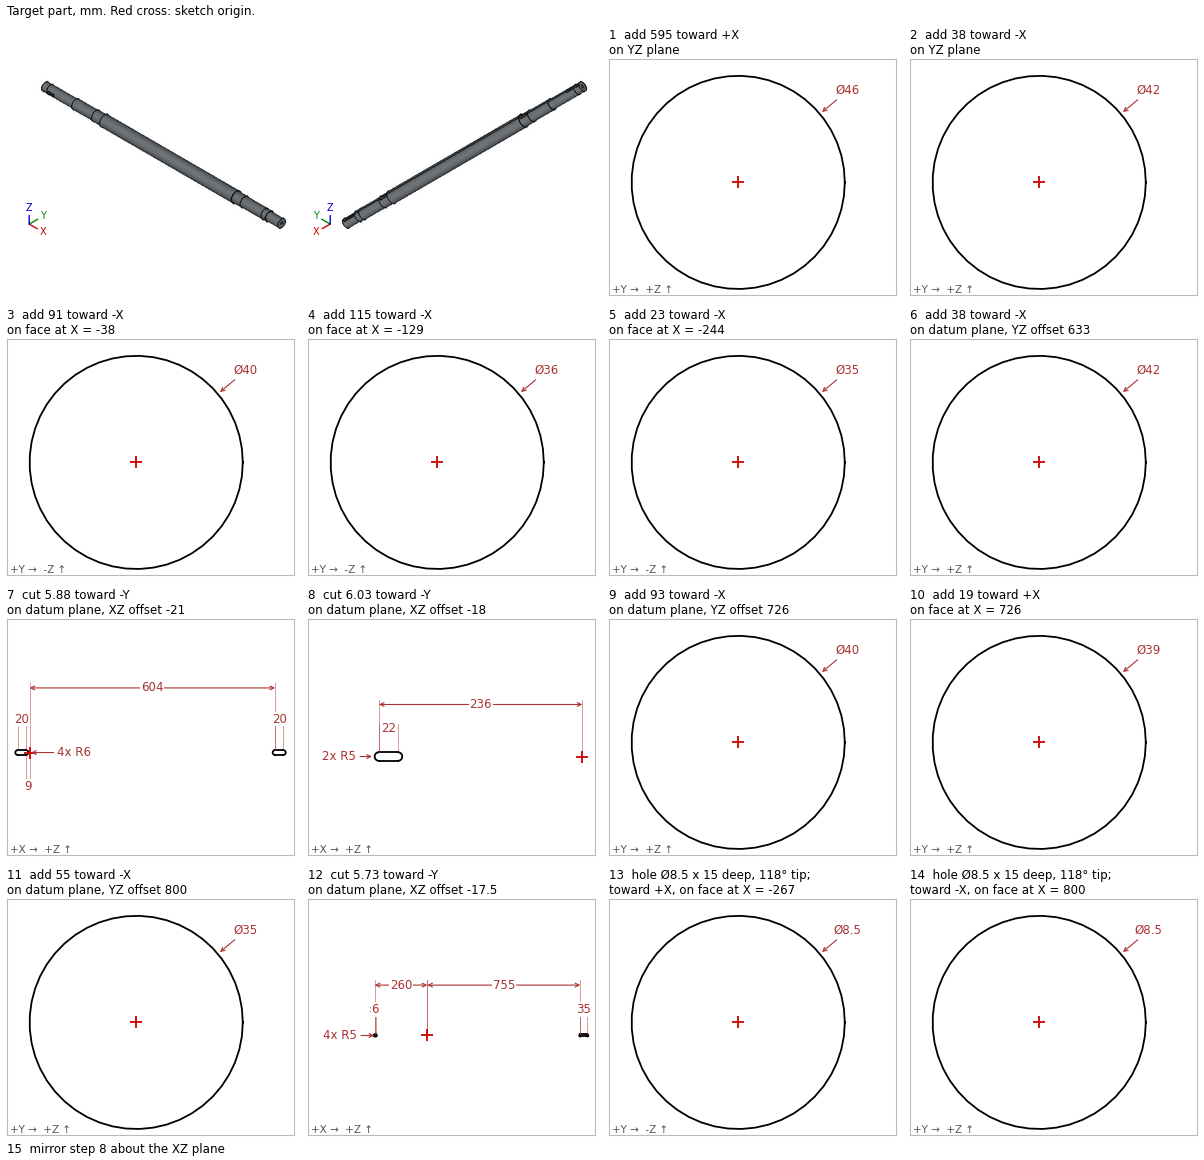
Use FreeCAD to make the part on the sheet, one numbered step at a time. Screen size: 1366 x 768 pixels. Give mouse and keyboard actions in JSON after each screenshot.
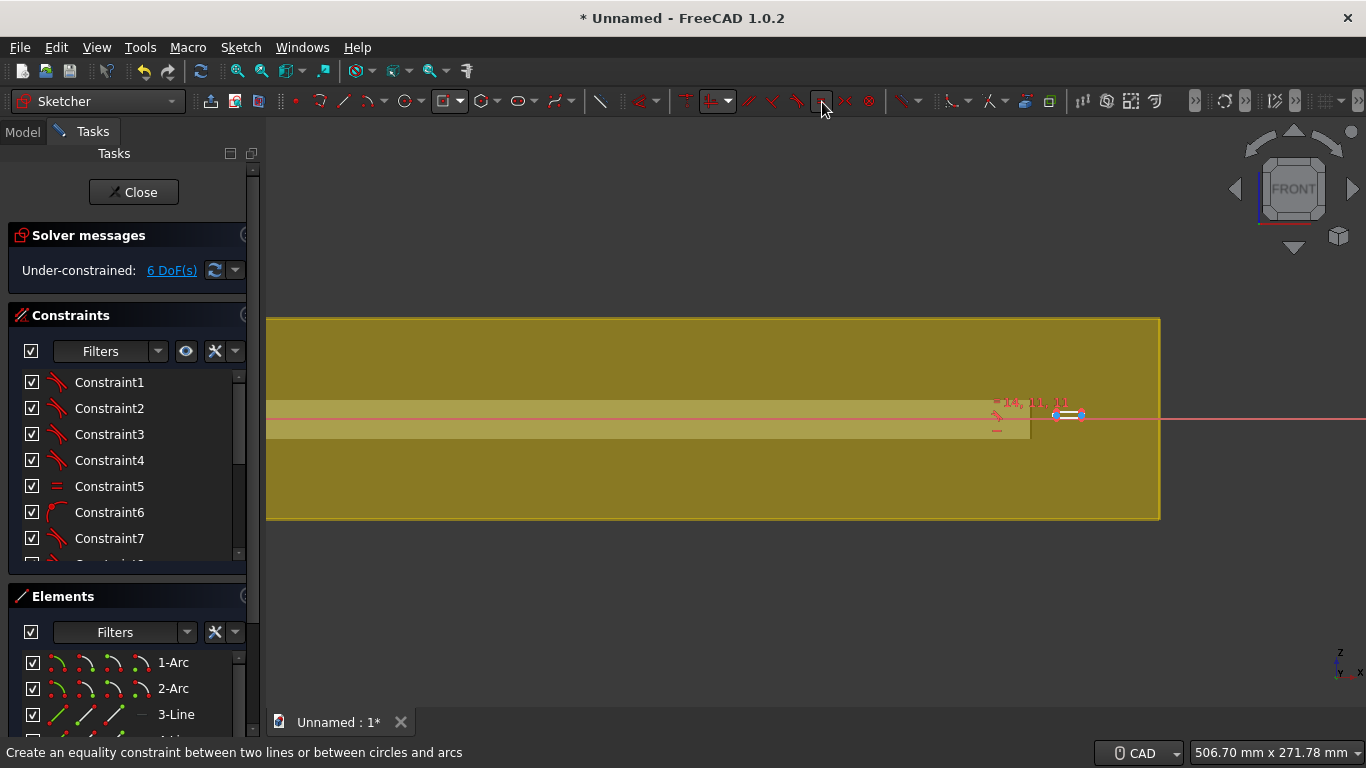
{"action": "scroll", "coordinate": [1056, 415], "scroll_direction": "up", "scroll_amount": 7}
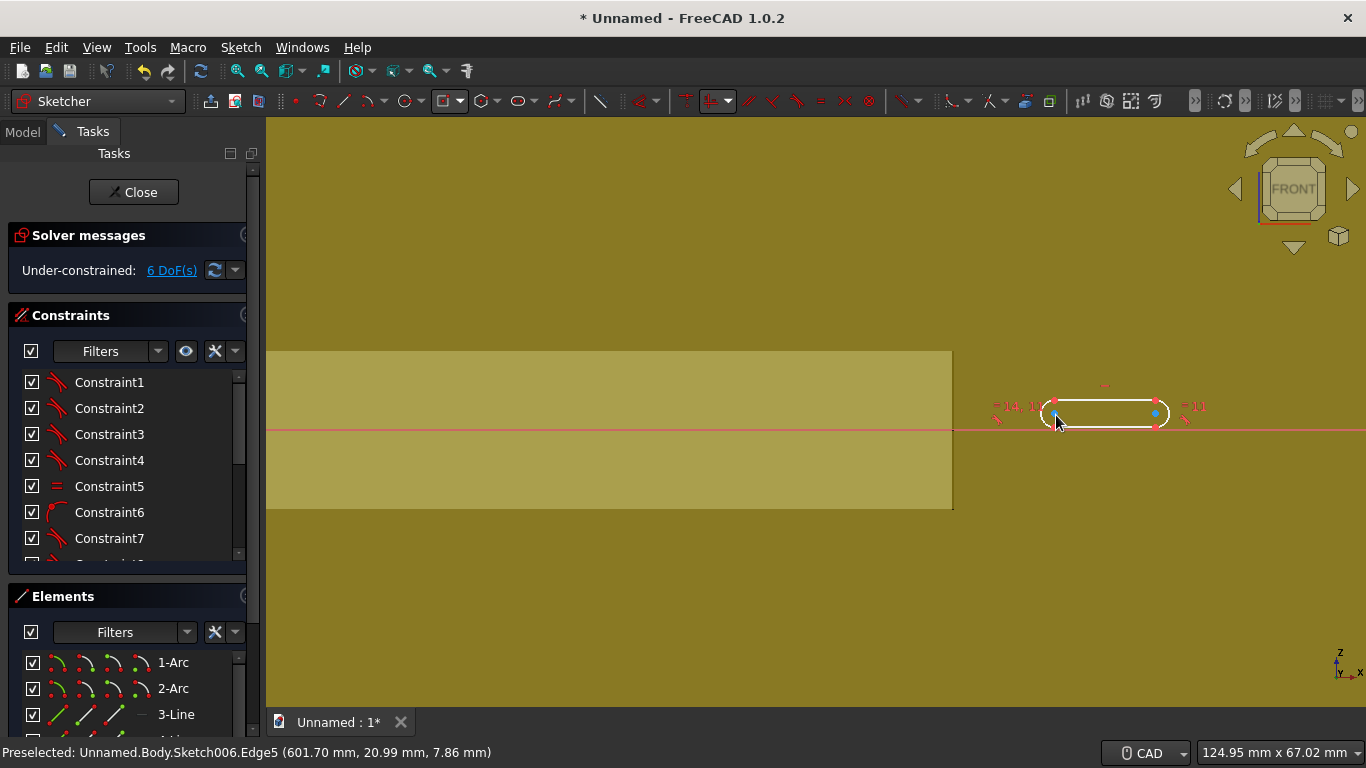
{"action": "left_click", "coordinate": [1055, 414]}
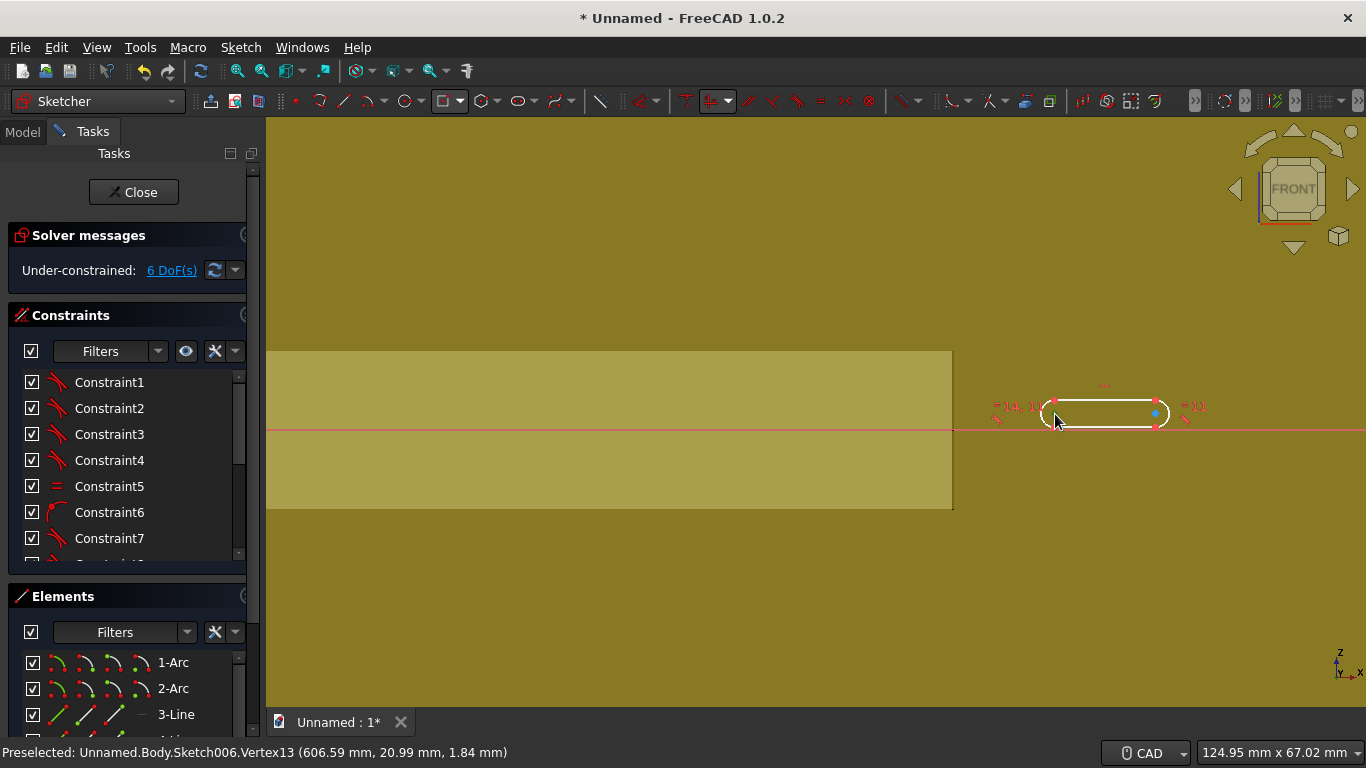
{"action": "left_click", "coordinate": [359, 430]}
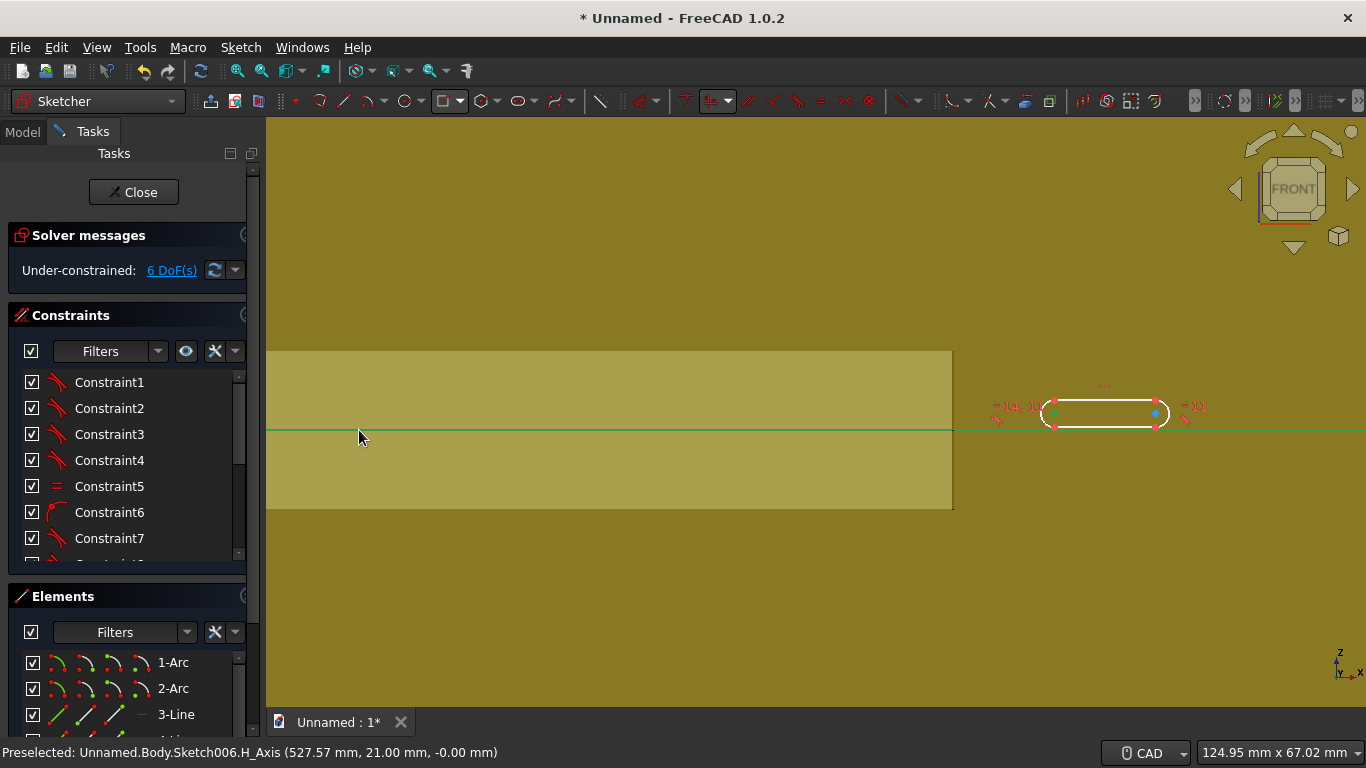
{"action": "key", "text": "c"}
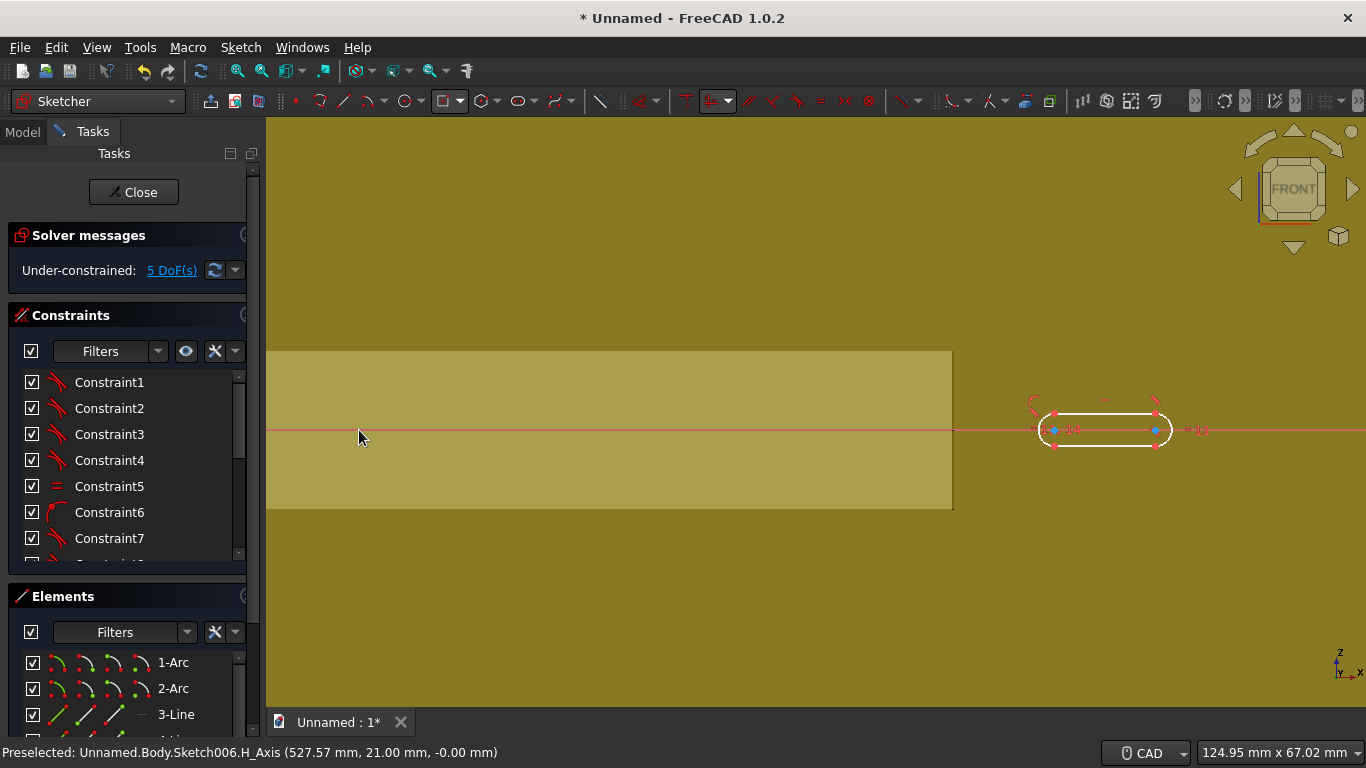
{"action": "scroll", "coordinate": [1048, 410], "scroll_direction": "down", "scroll_amount": 11}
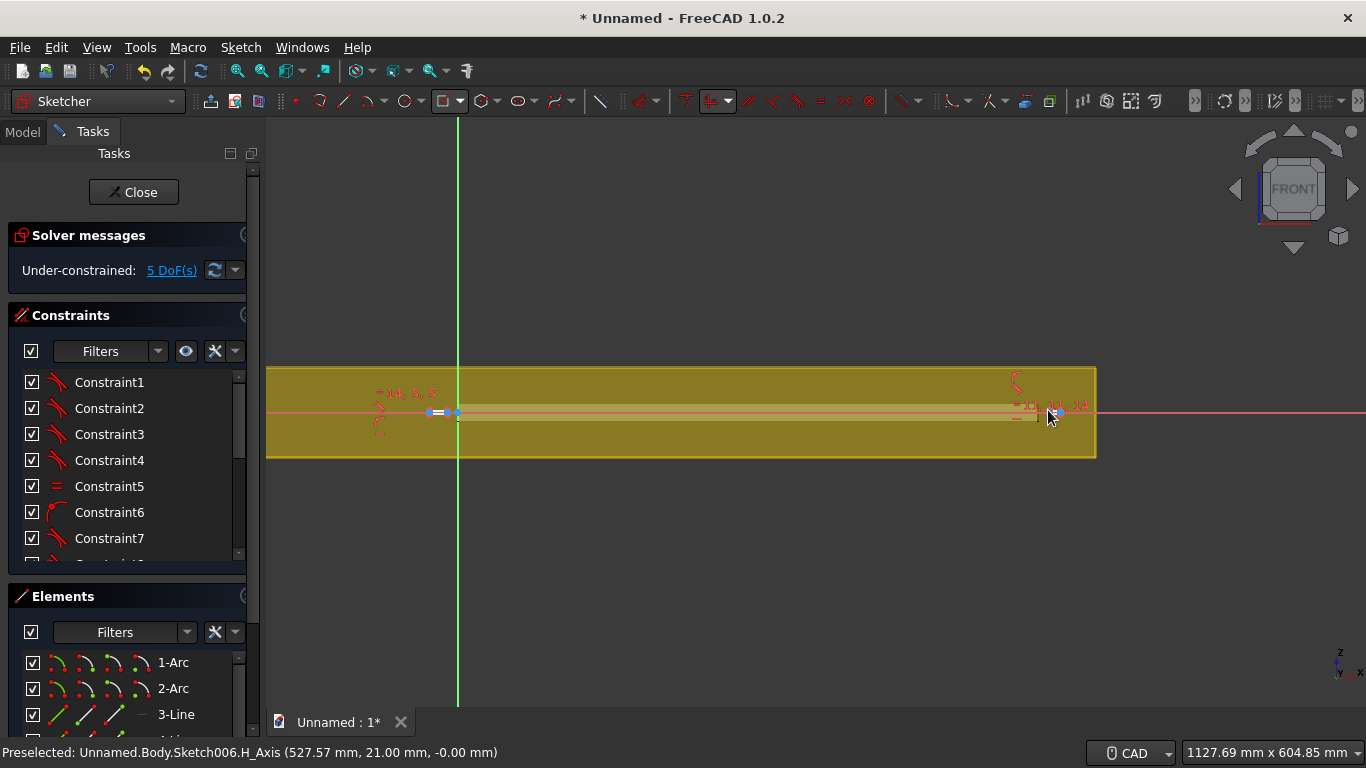
{"action": "scroll", "coordinate": [429, 412], "scroll_direction": "up", "scroll_amount": 13}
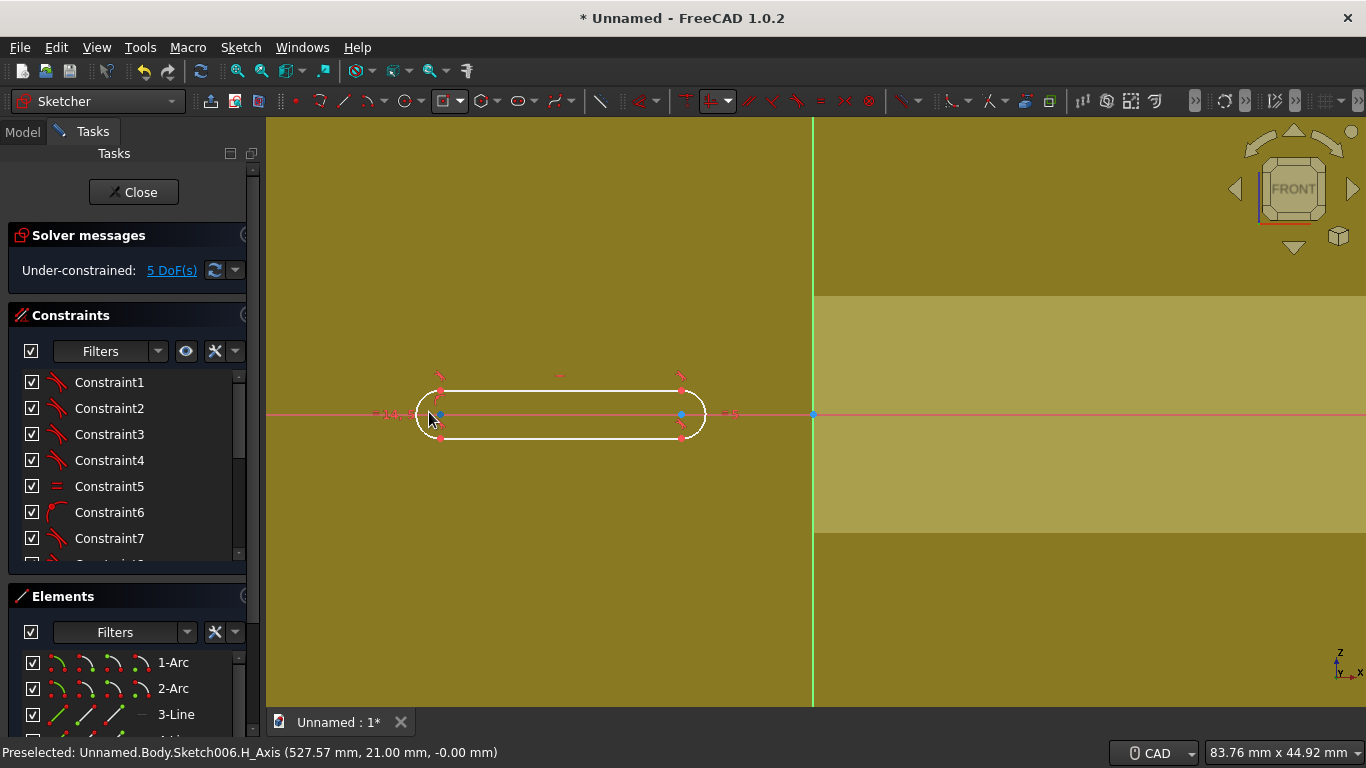
{"action": "left_click", "coordinate": [421, 401]}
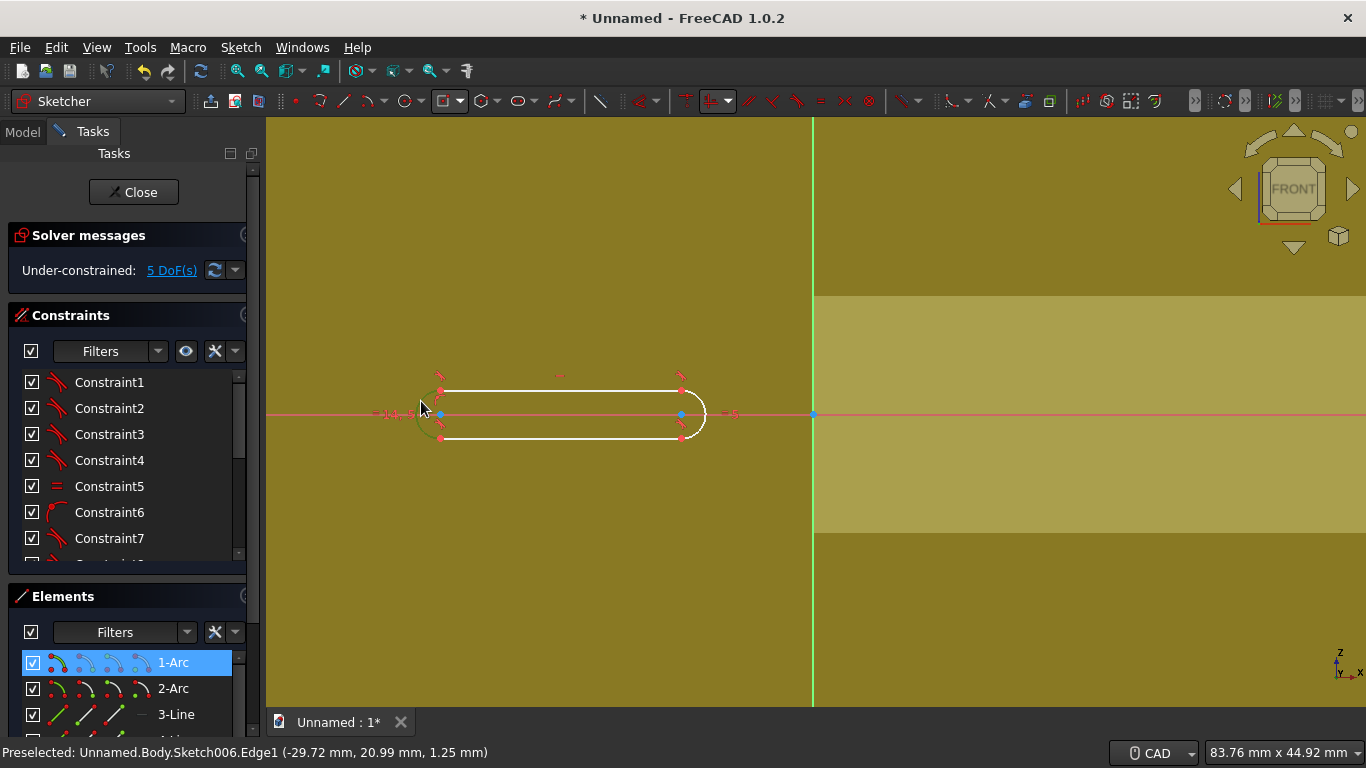
{"action": "left_click", "coordinate": [658, 102]}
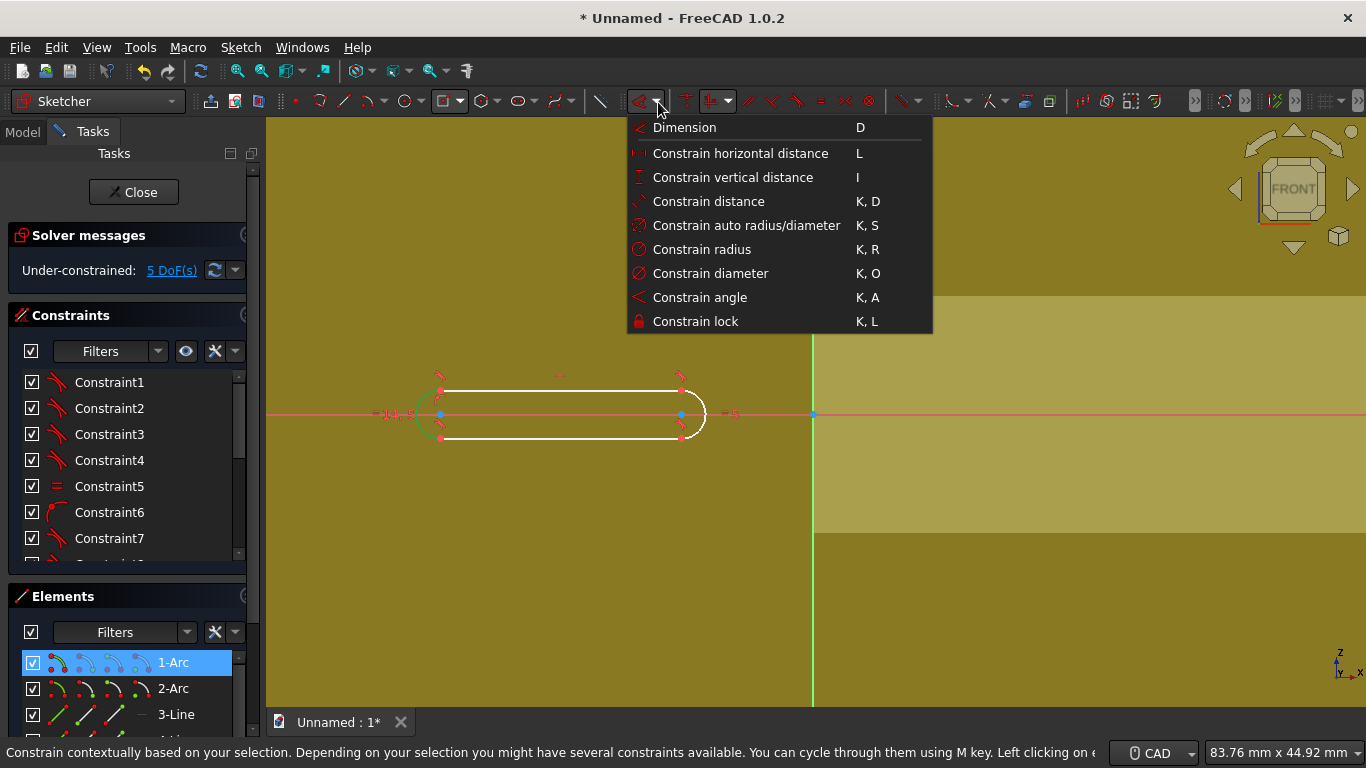
{"action": "left_click", "coordinate": [780, 249]}